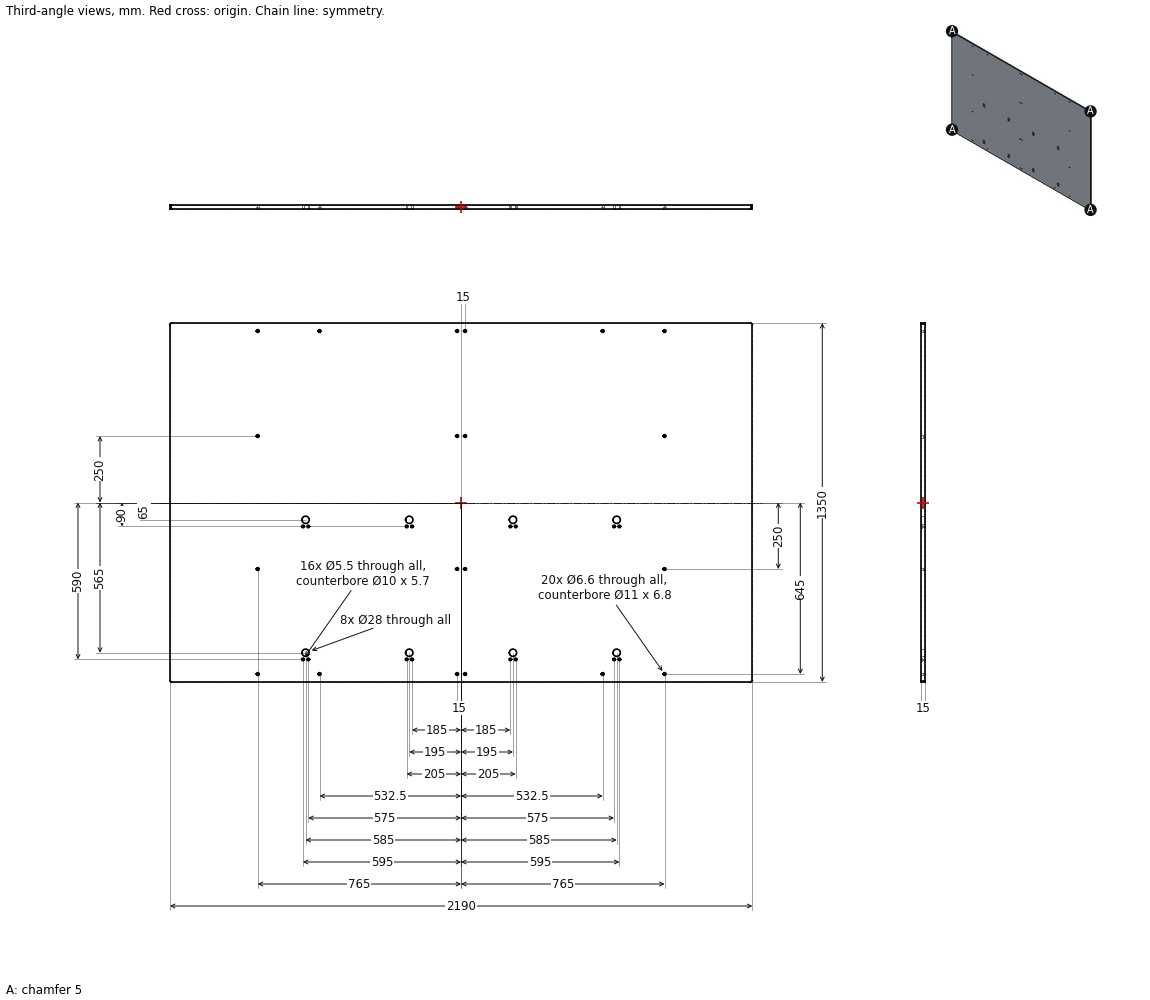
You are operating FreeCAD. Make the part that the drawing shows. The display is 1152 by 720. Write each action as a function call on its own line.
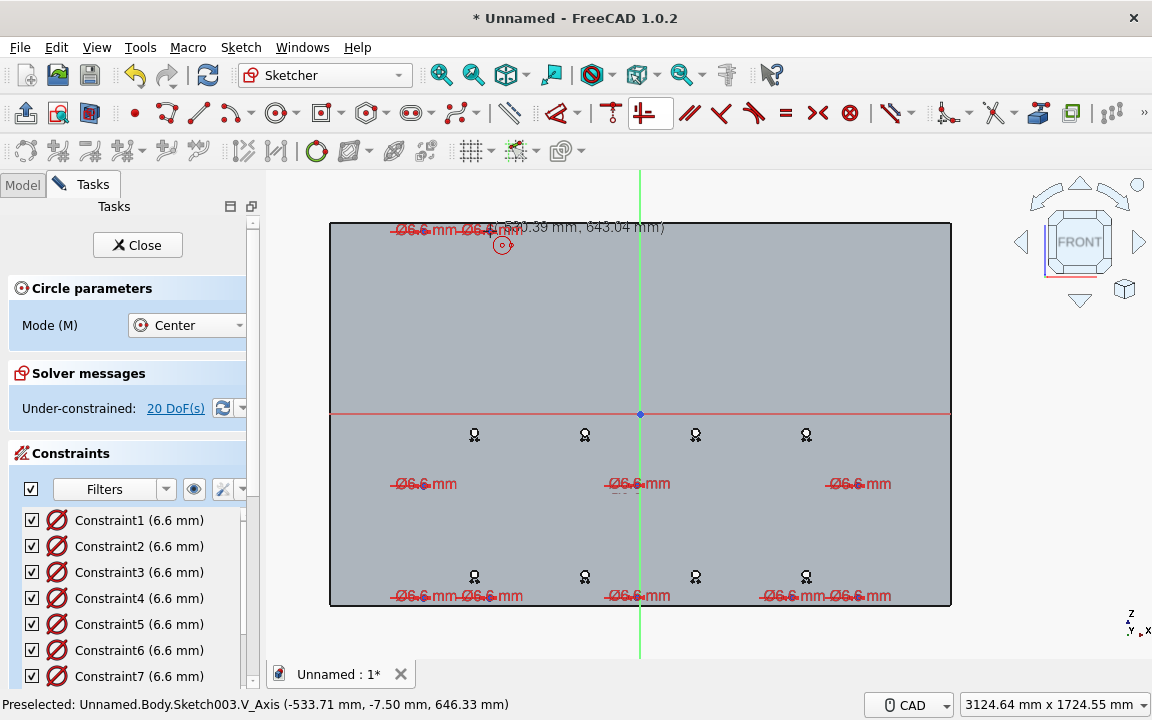
scroll(423, 343, up, 16)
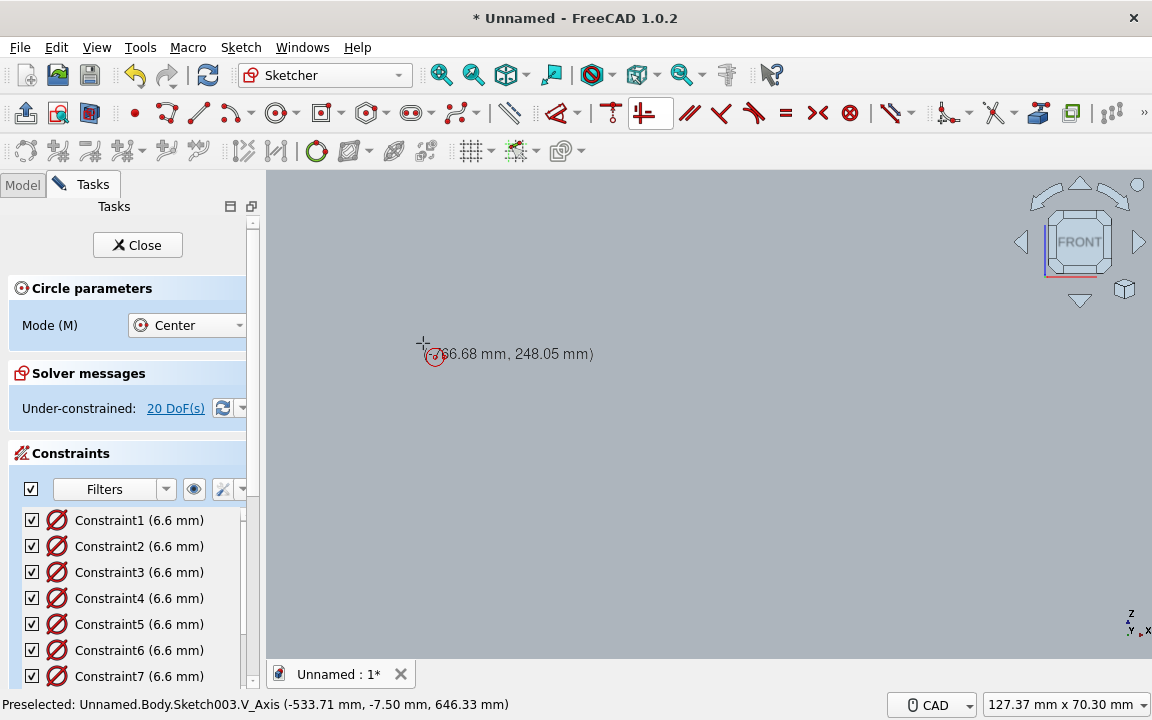
scroll(423, 344, down, 16)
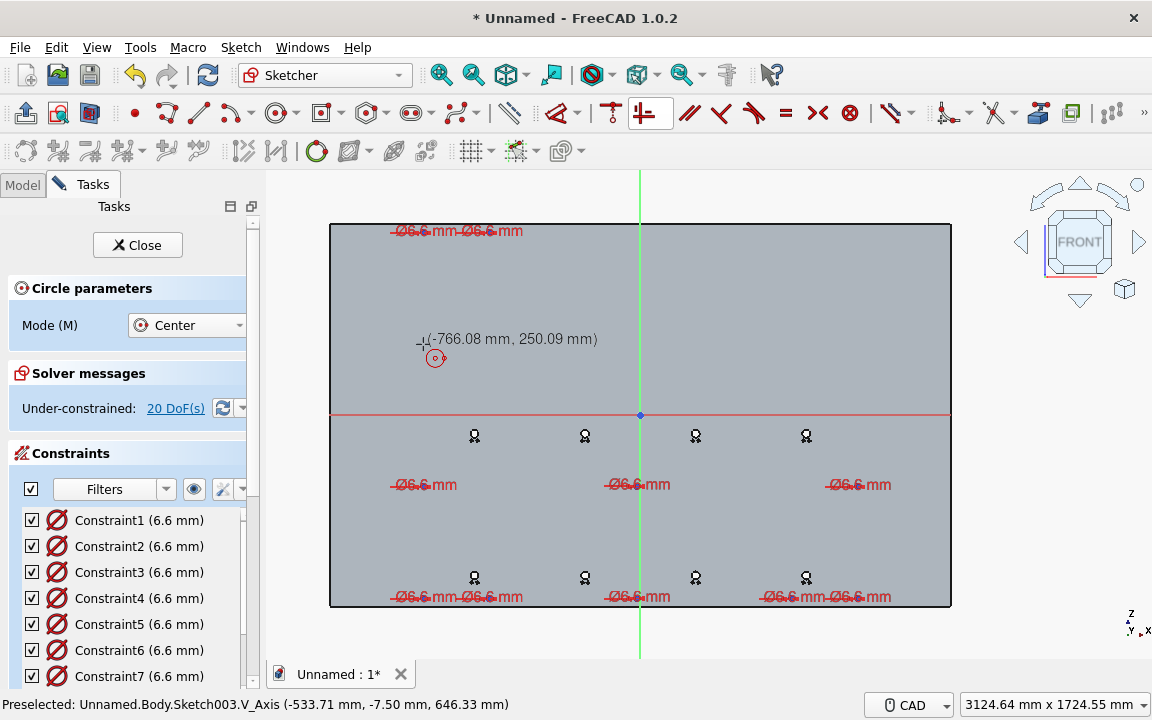
click(423, 344)
move(424, 344)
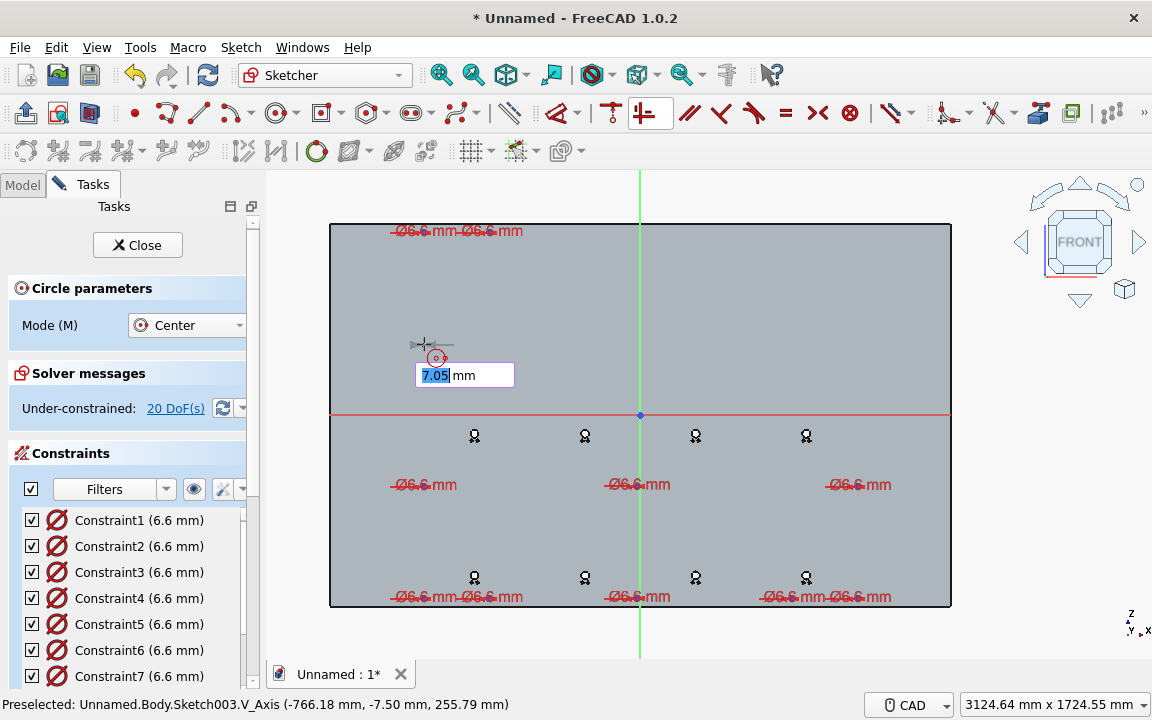
text(6.6)
key(Return)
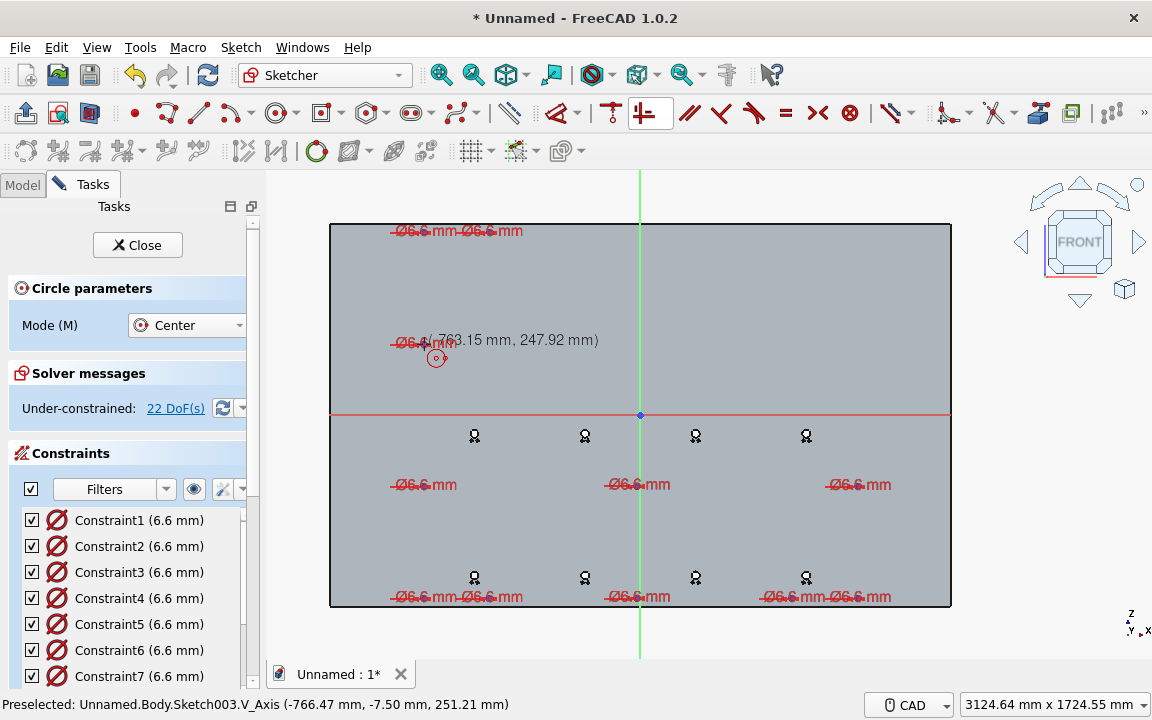
scroll(636, 344, up, 16)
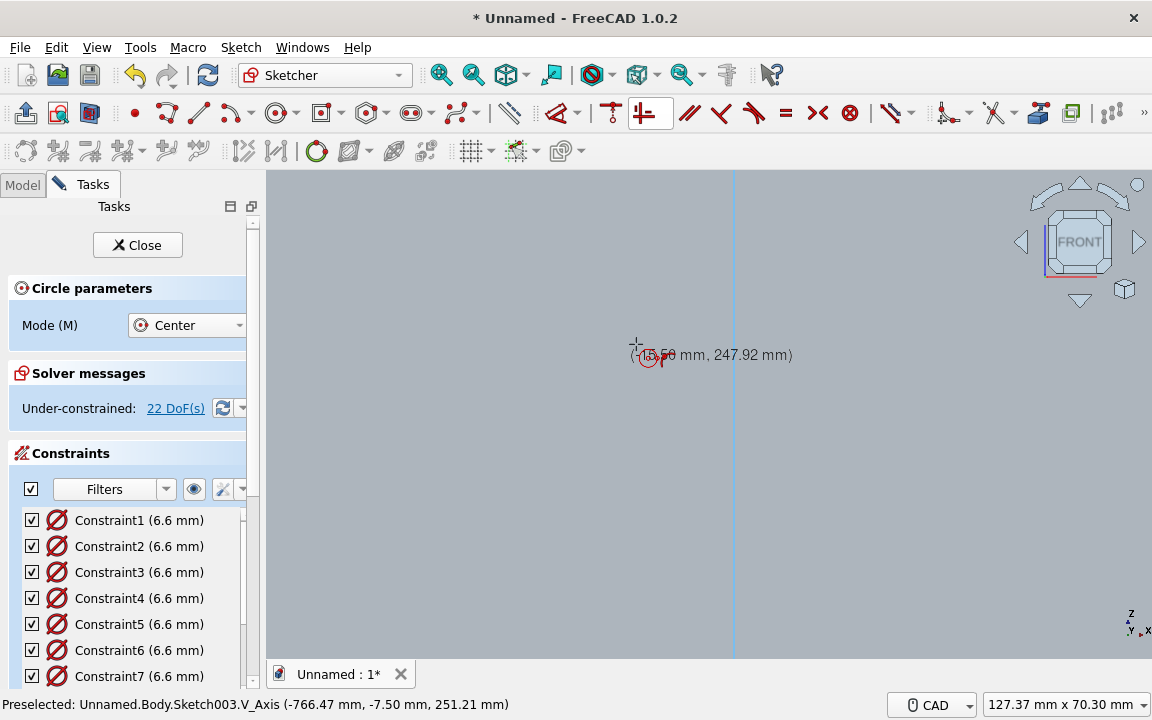
scroll(637, 344, down, 16)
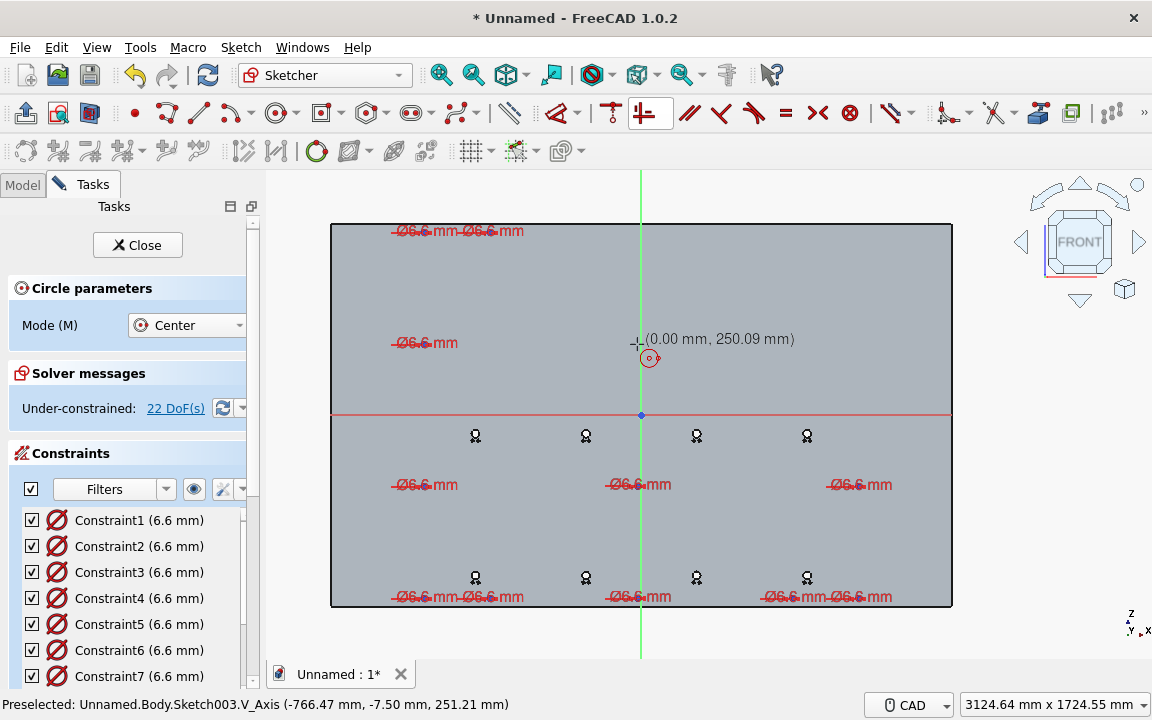
scroll(637, 344, up, 7)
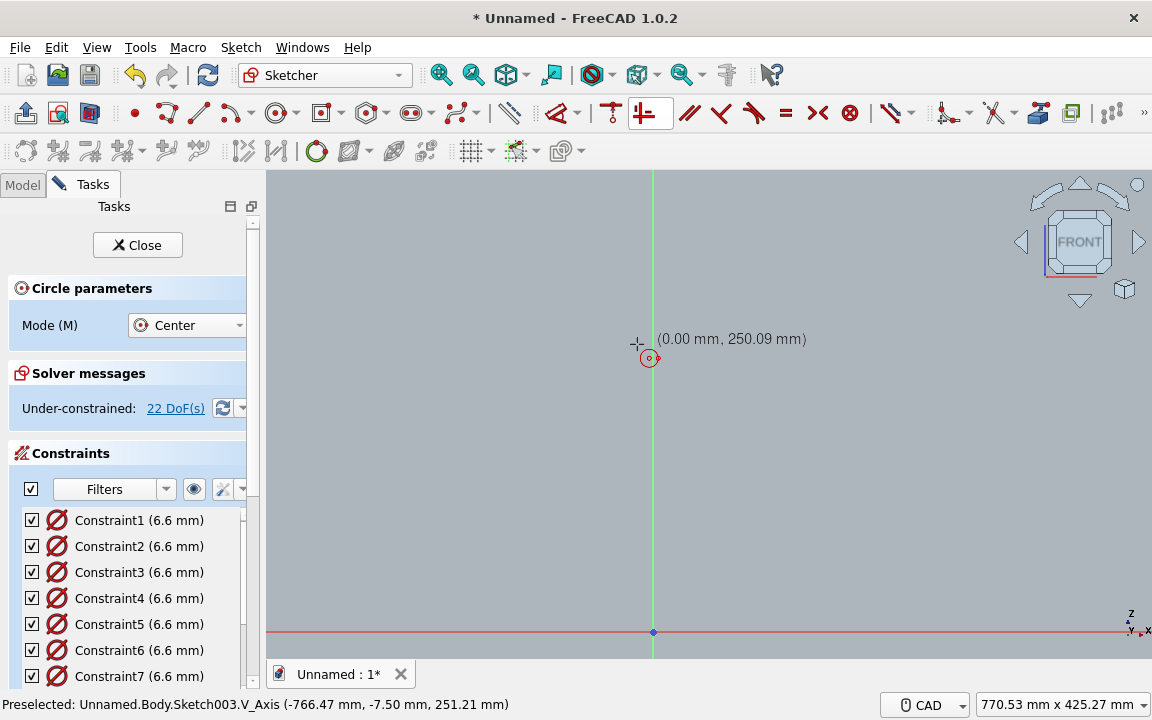
click(636, 345)
move(639, 342)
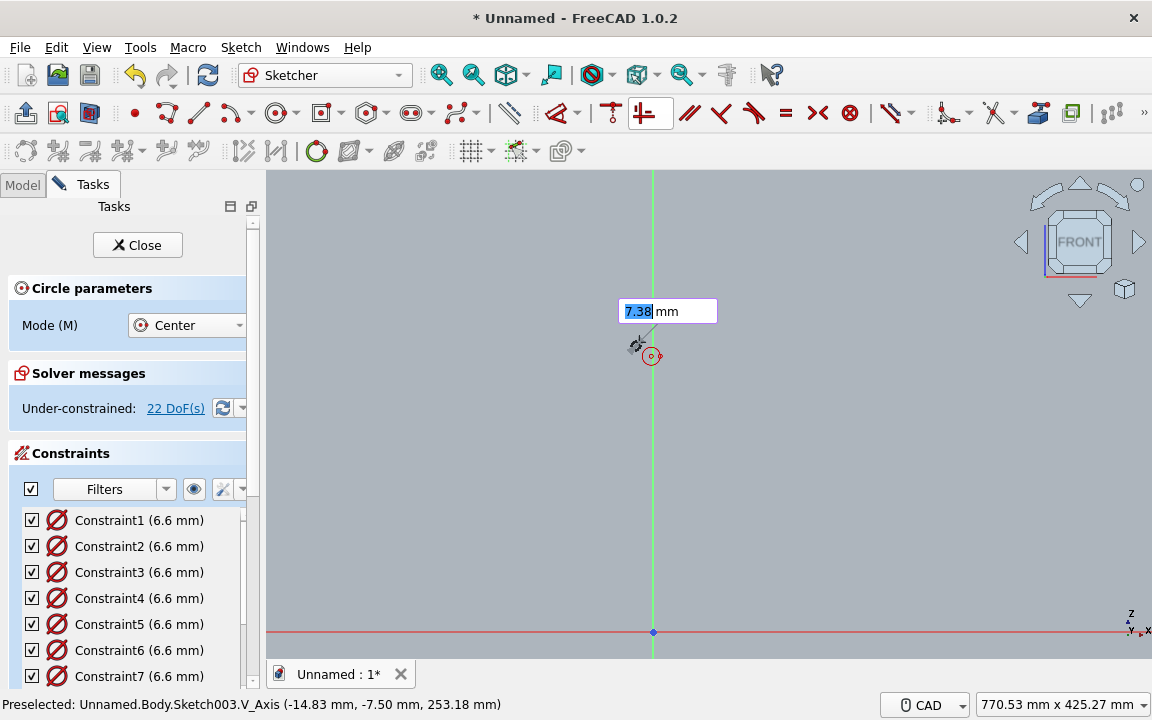
text(6.6)
key(Return)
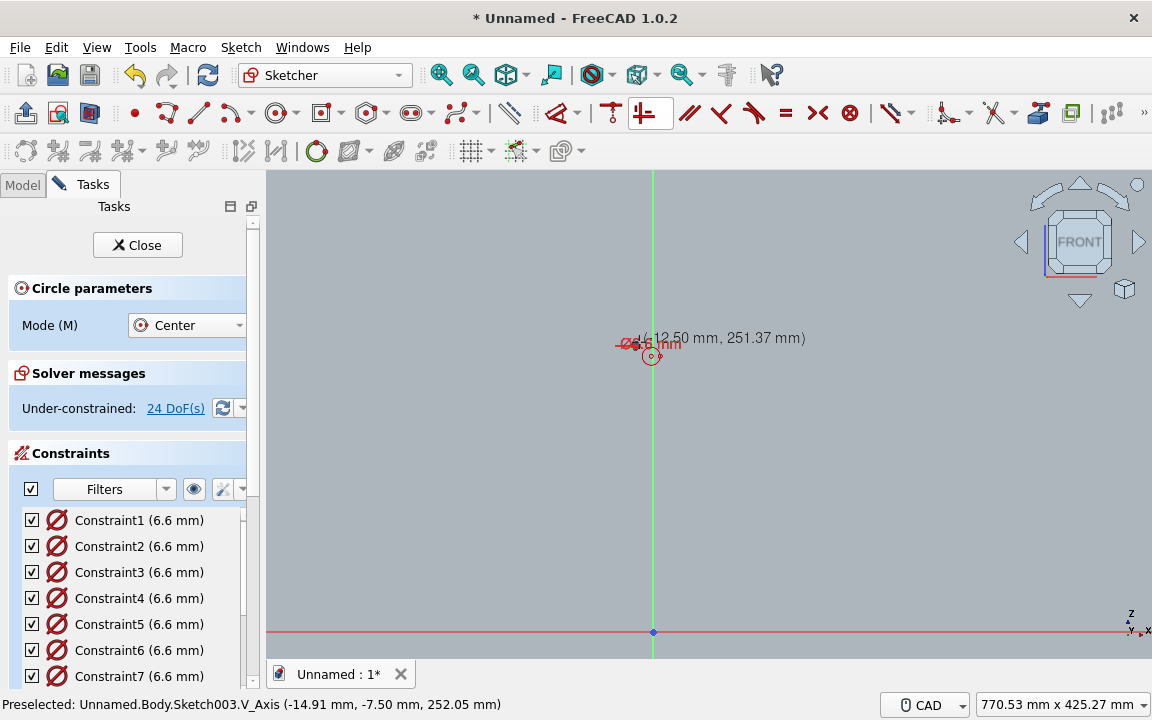
scroll(637, 359, down, 8)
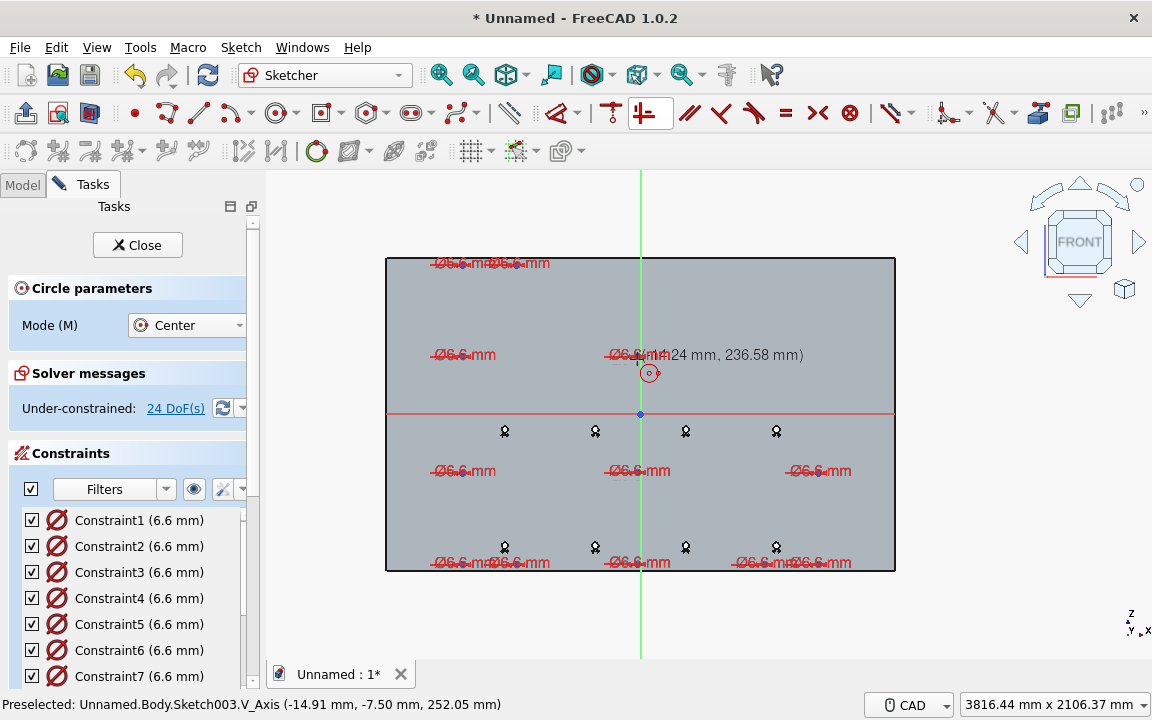
scroll(637, 265, up, 17)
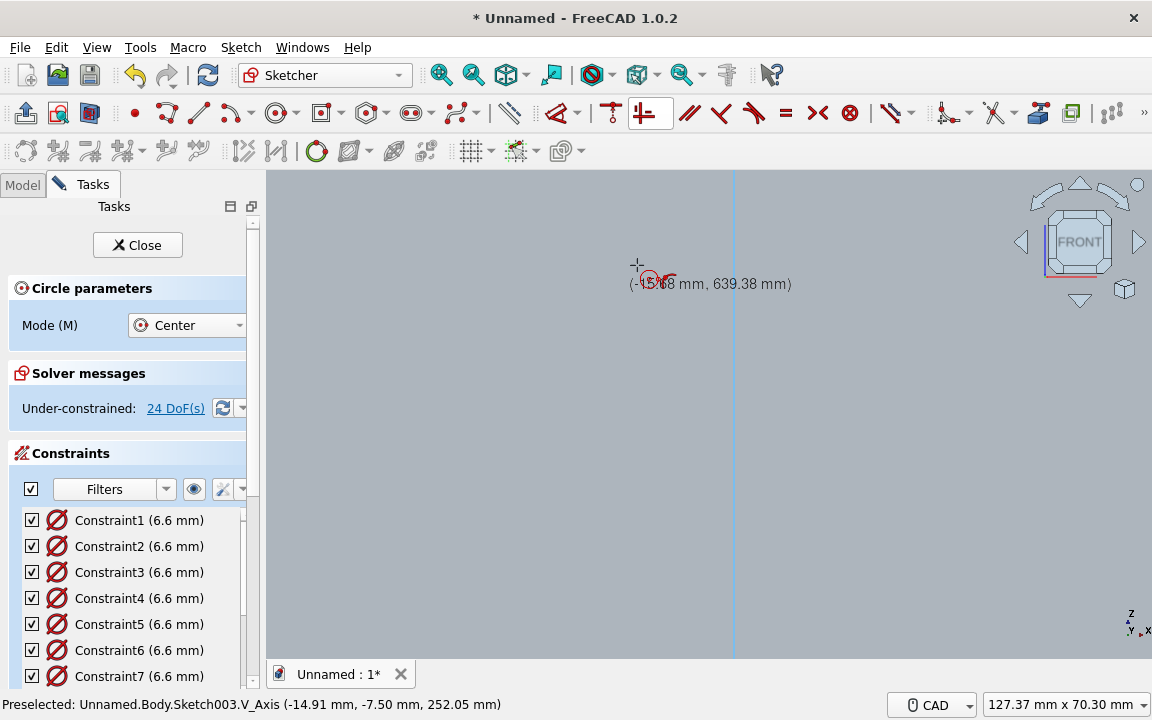
scroll(637, 231, down, 16)